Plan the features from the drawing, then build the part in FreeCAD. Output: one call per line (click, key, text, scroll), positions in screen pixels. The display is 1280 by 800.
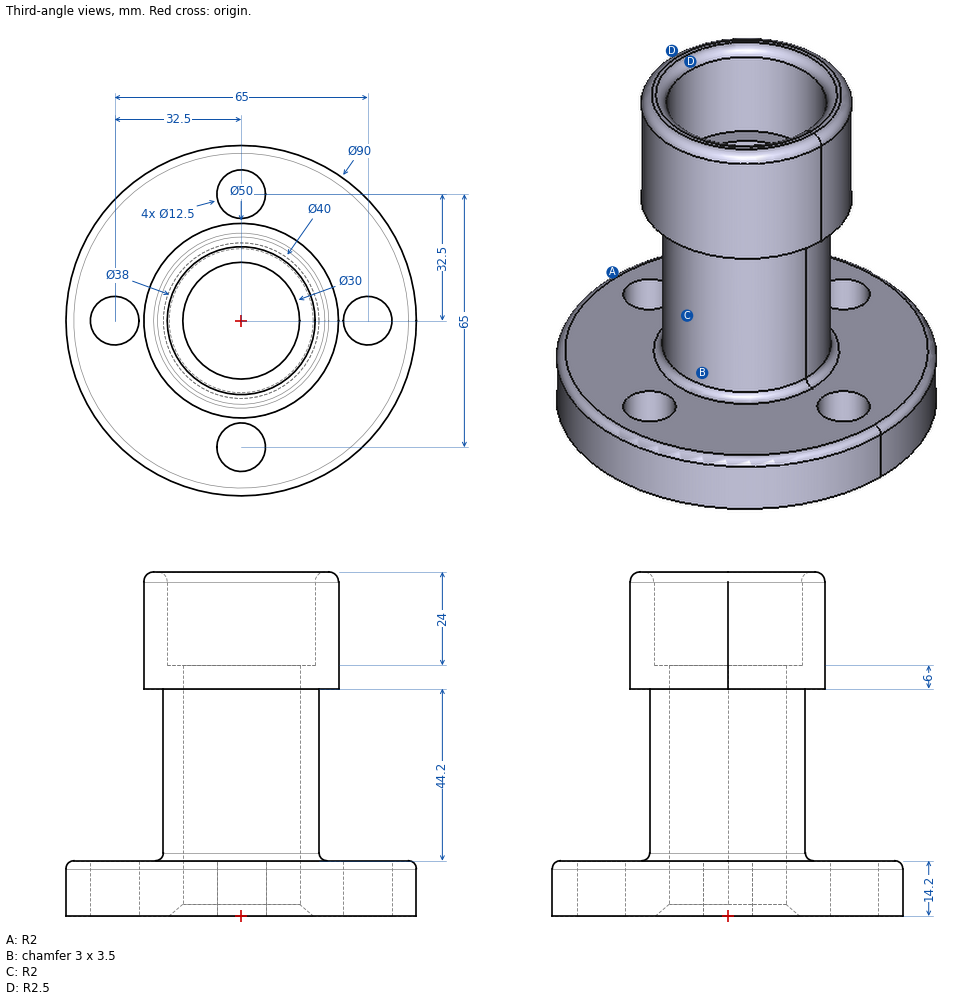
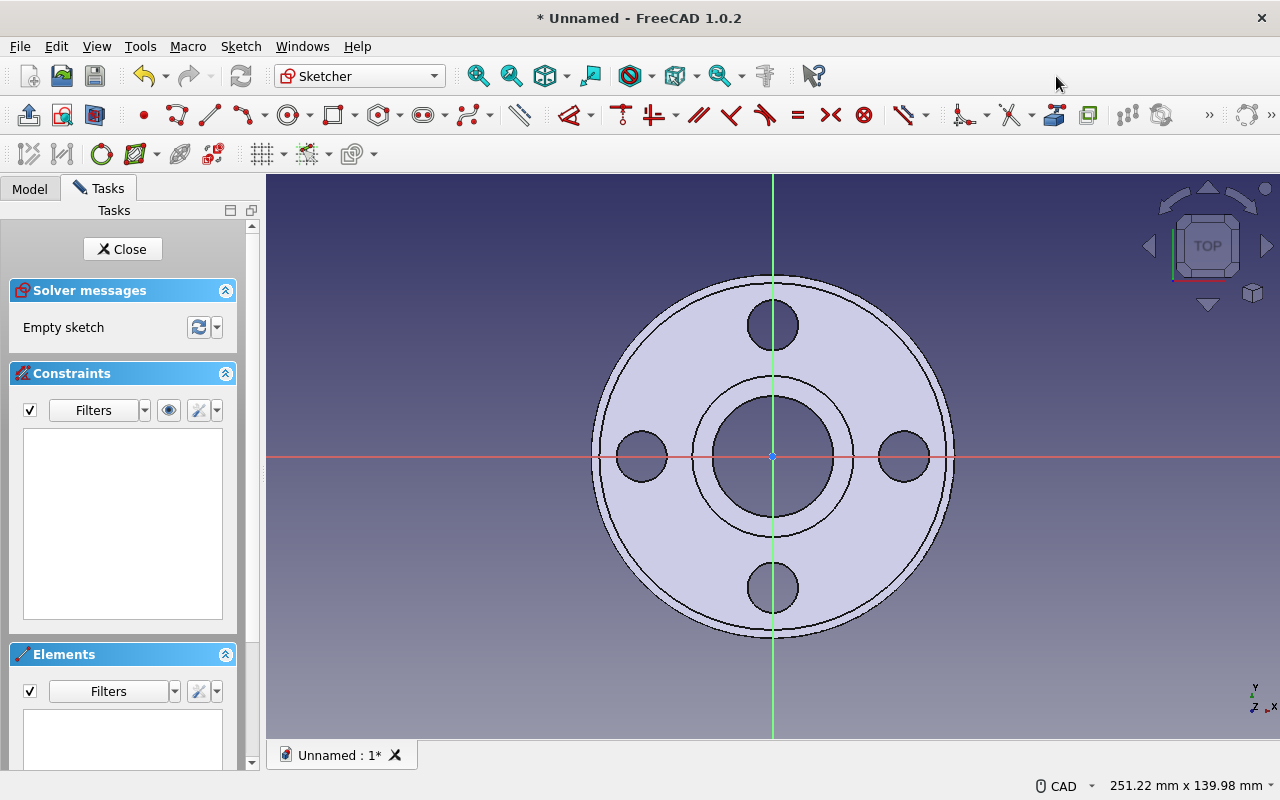
scroll(856, 456, up, 3)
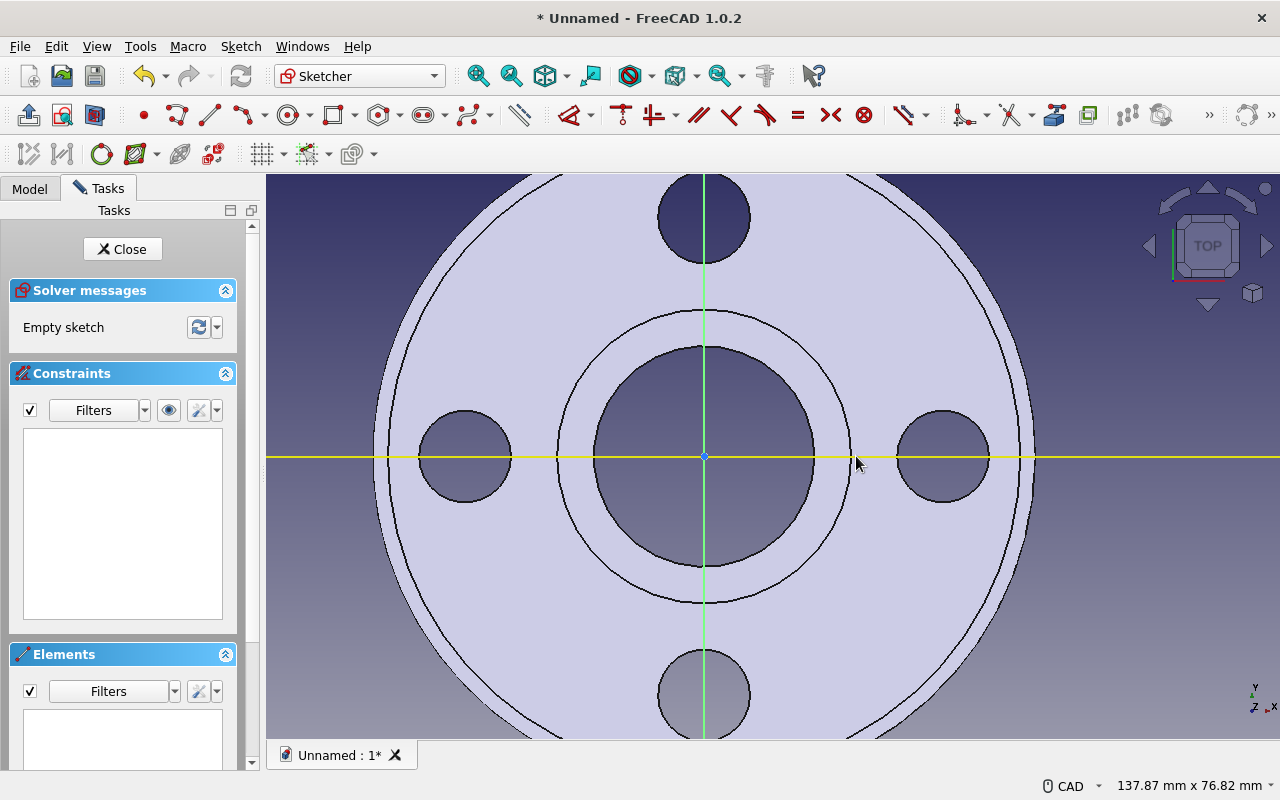
click(288, 116)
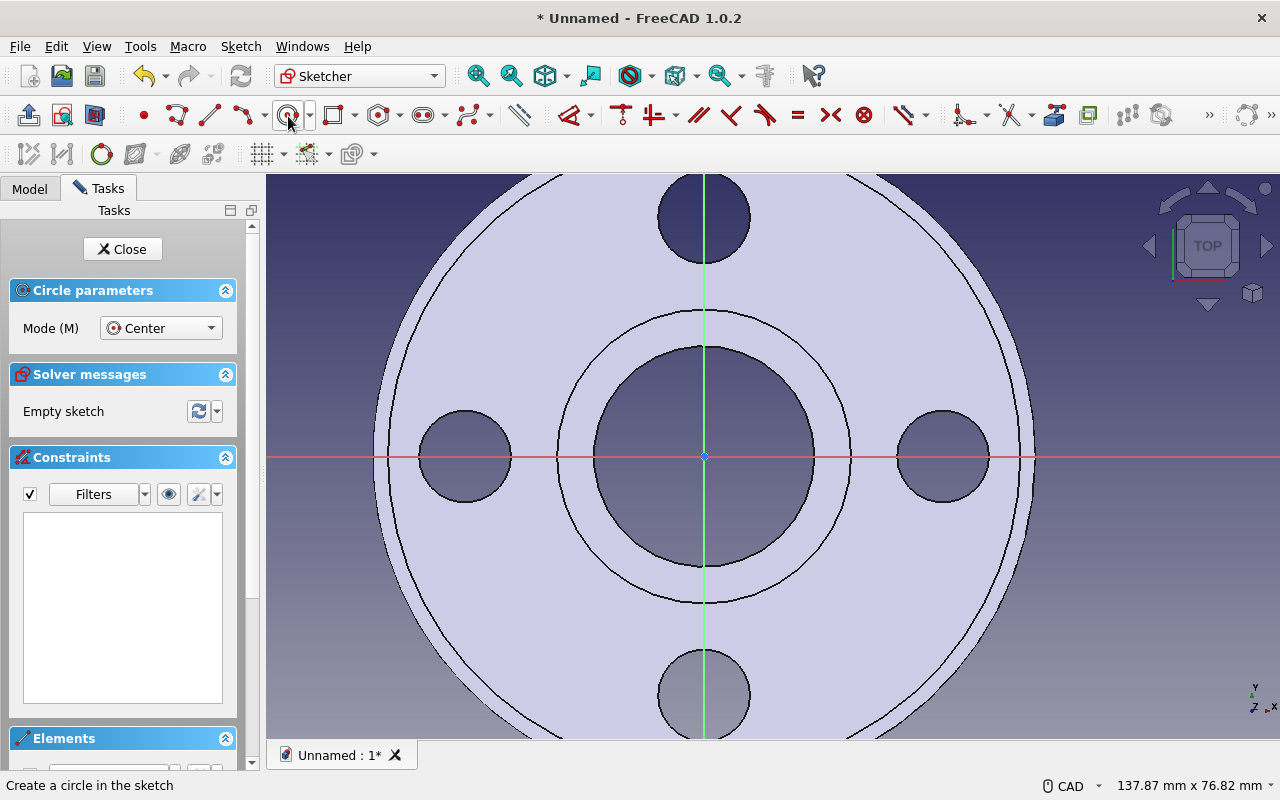
click(704, 456)
move(834, 326)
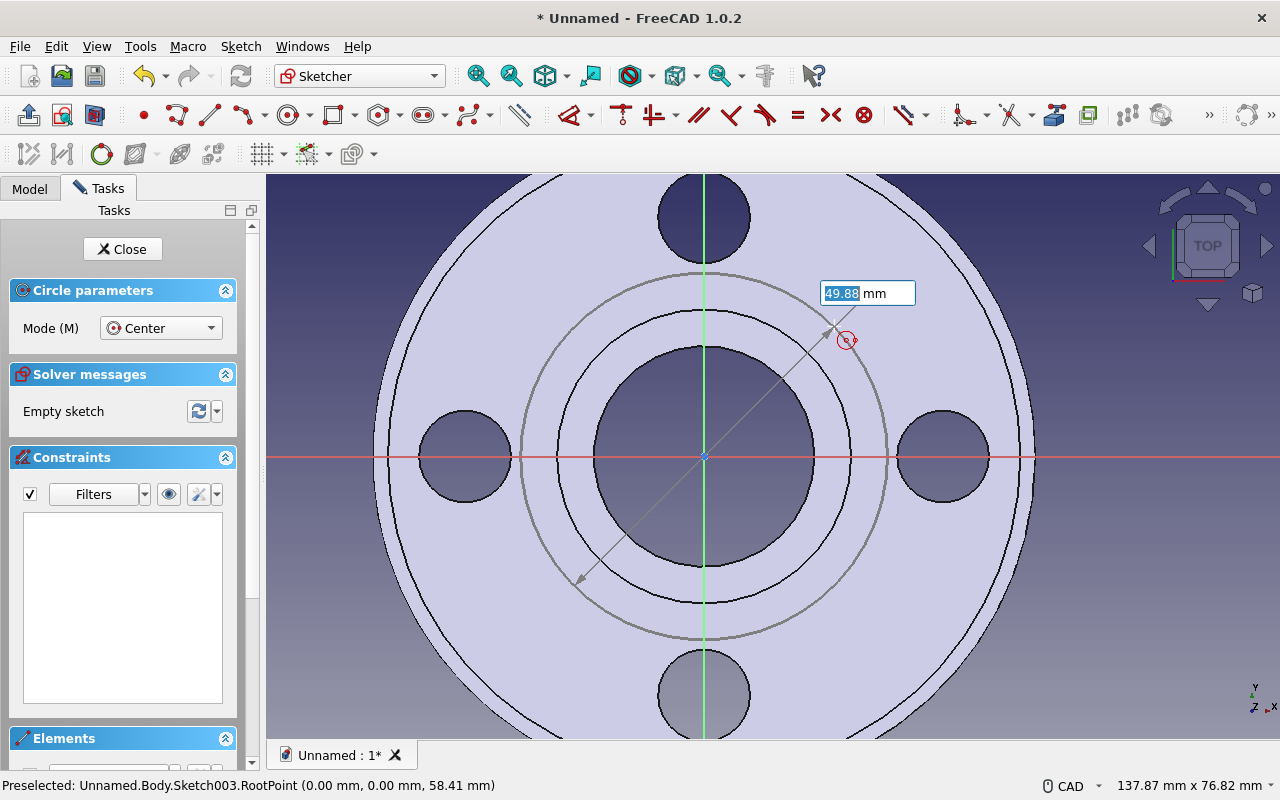
text(50)
key(Return)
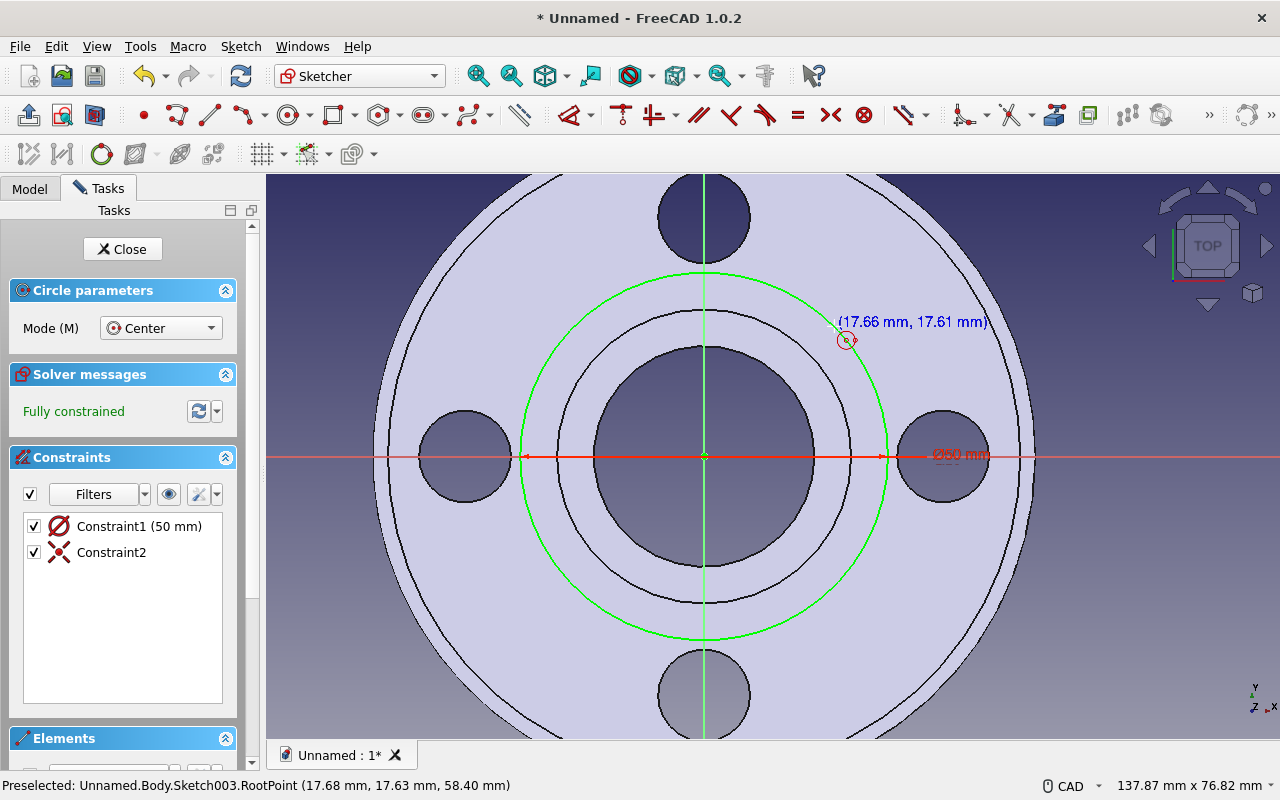
click(704, 456)
move(782, 378)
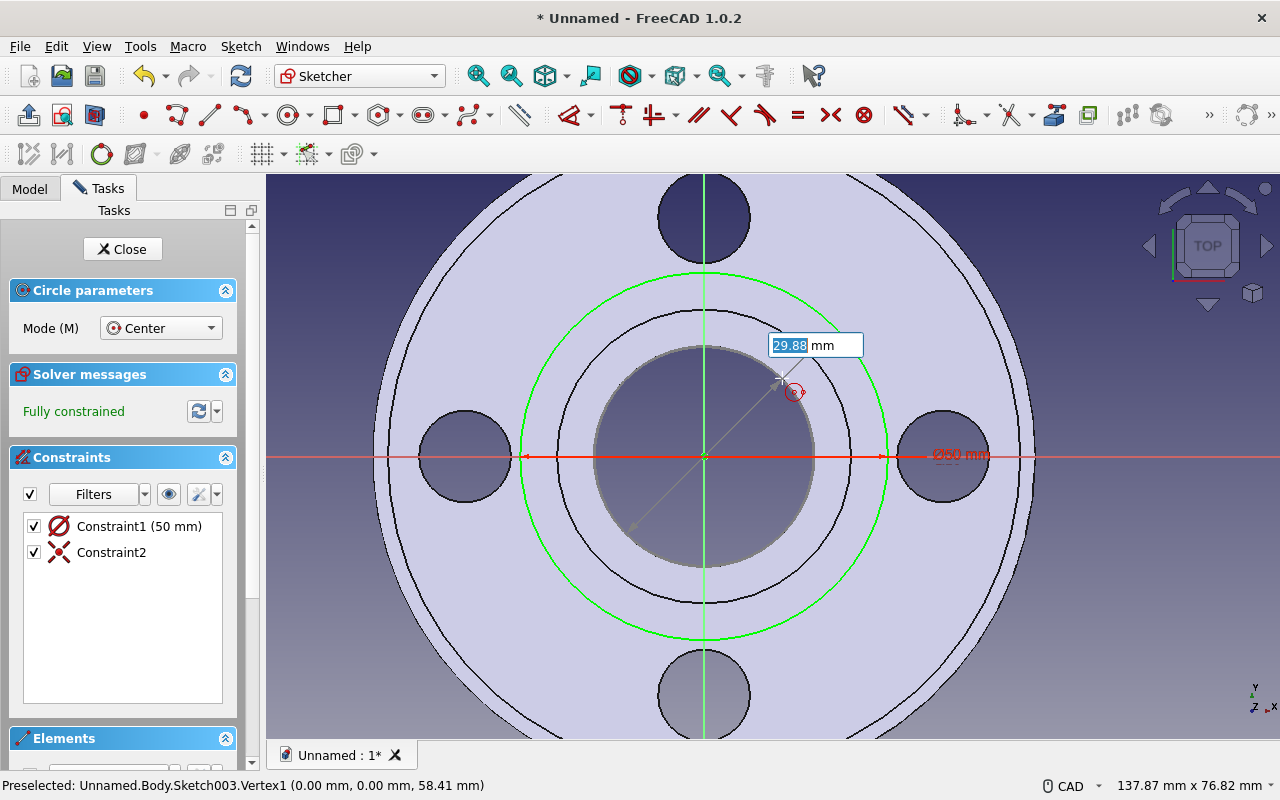
text(30)
key(Return)
key(Escape)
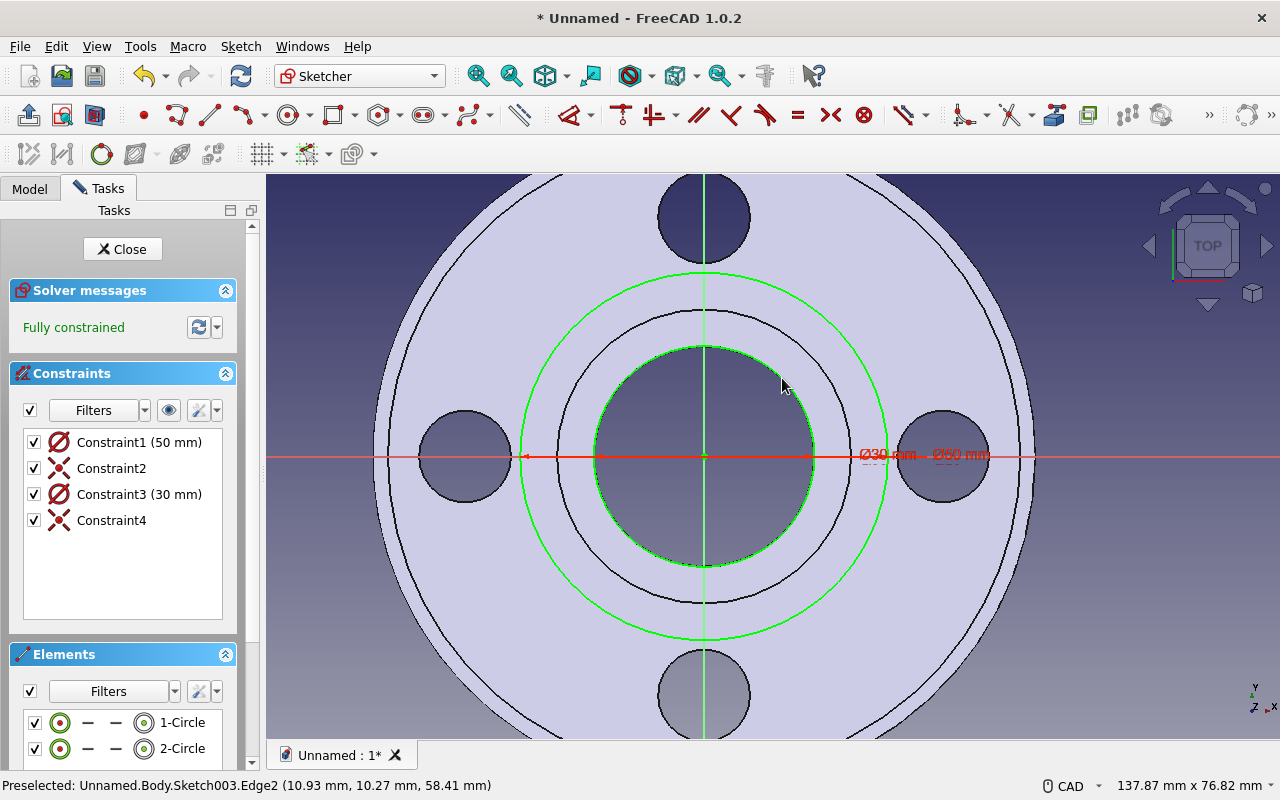
click(123, 249)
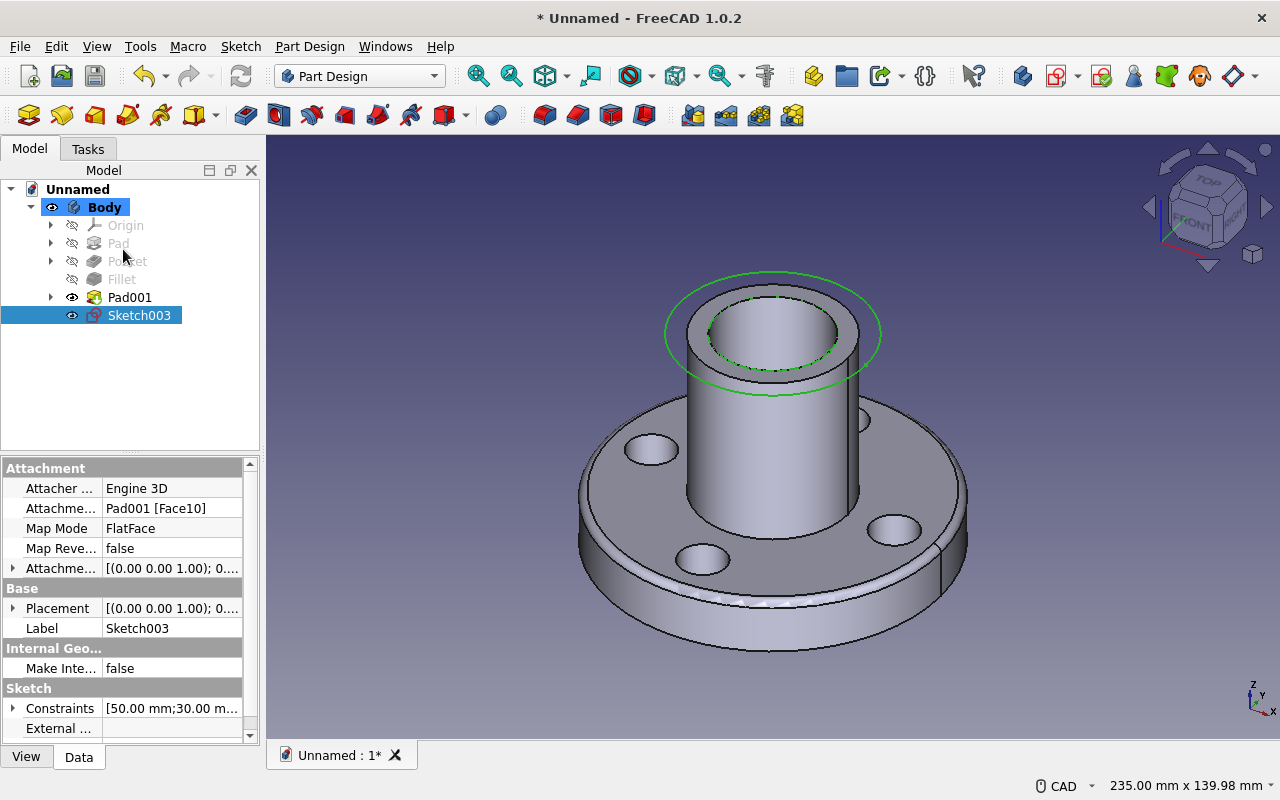
click(29, 116)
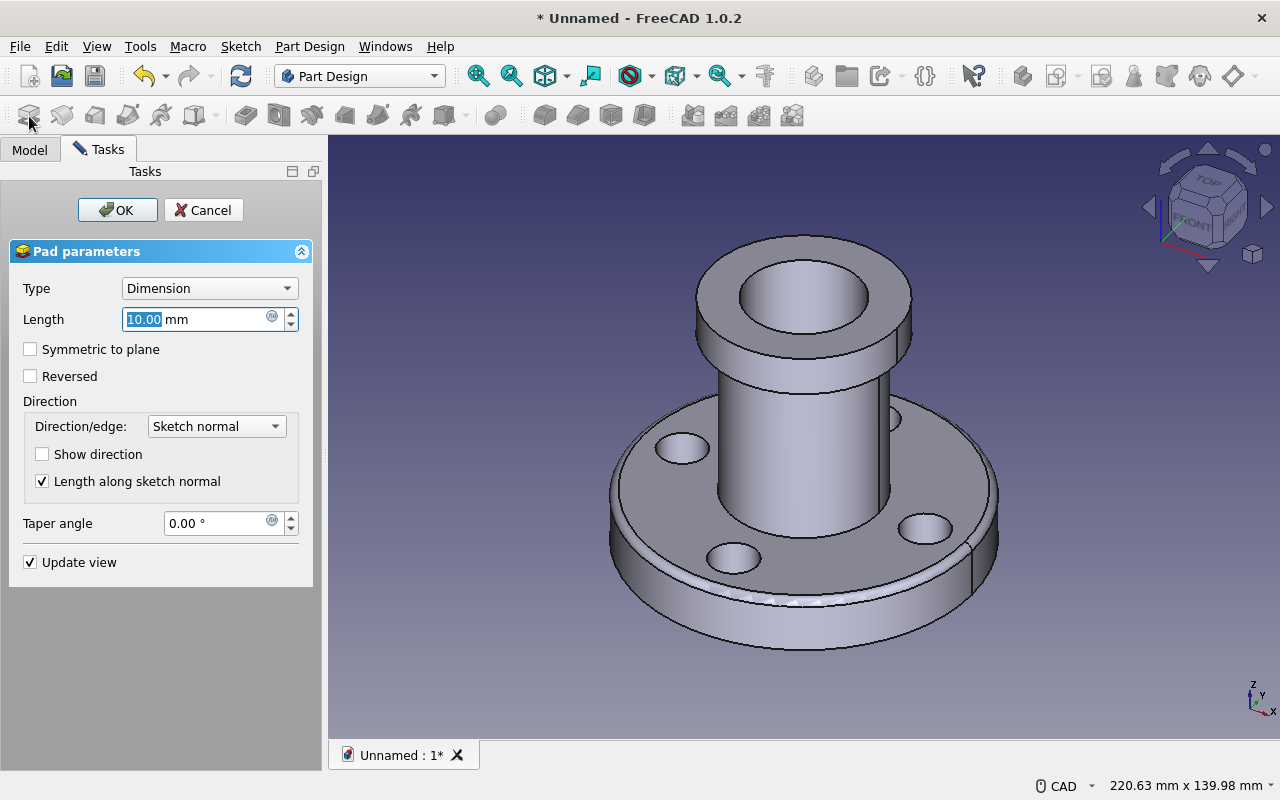
text(6)
key(Tab)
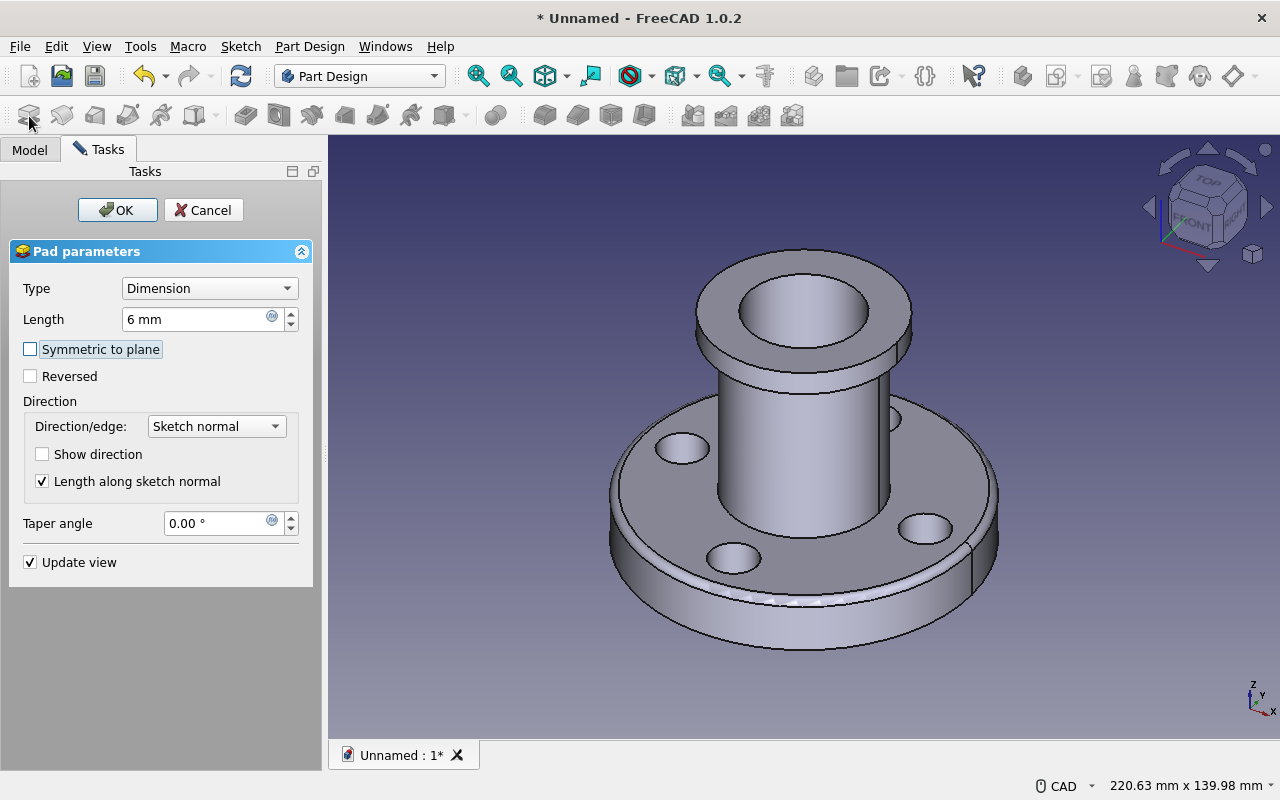
click(118, 210)